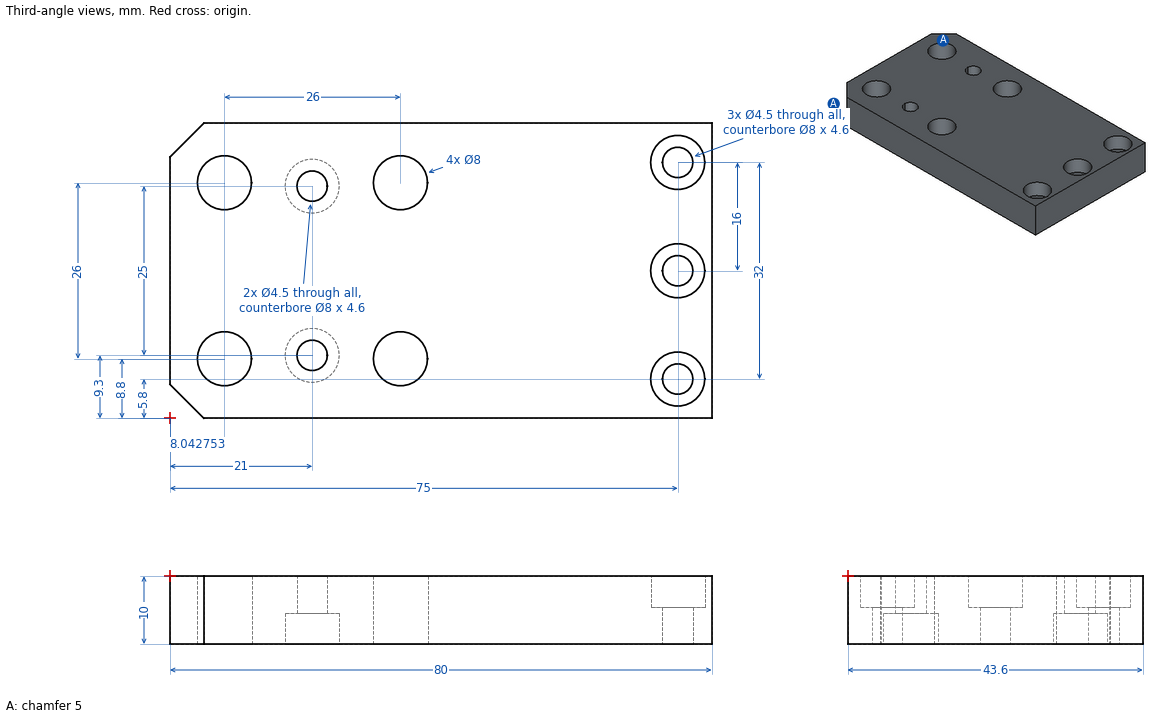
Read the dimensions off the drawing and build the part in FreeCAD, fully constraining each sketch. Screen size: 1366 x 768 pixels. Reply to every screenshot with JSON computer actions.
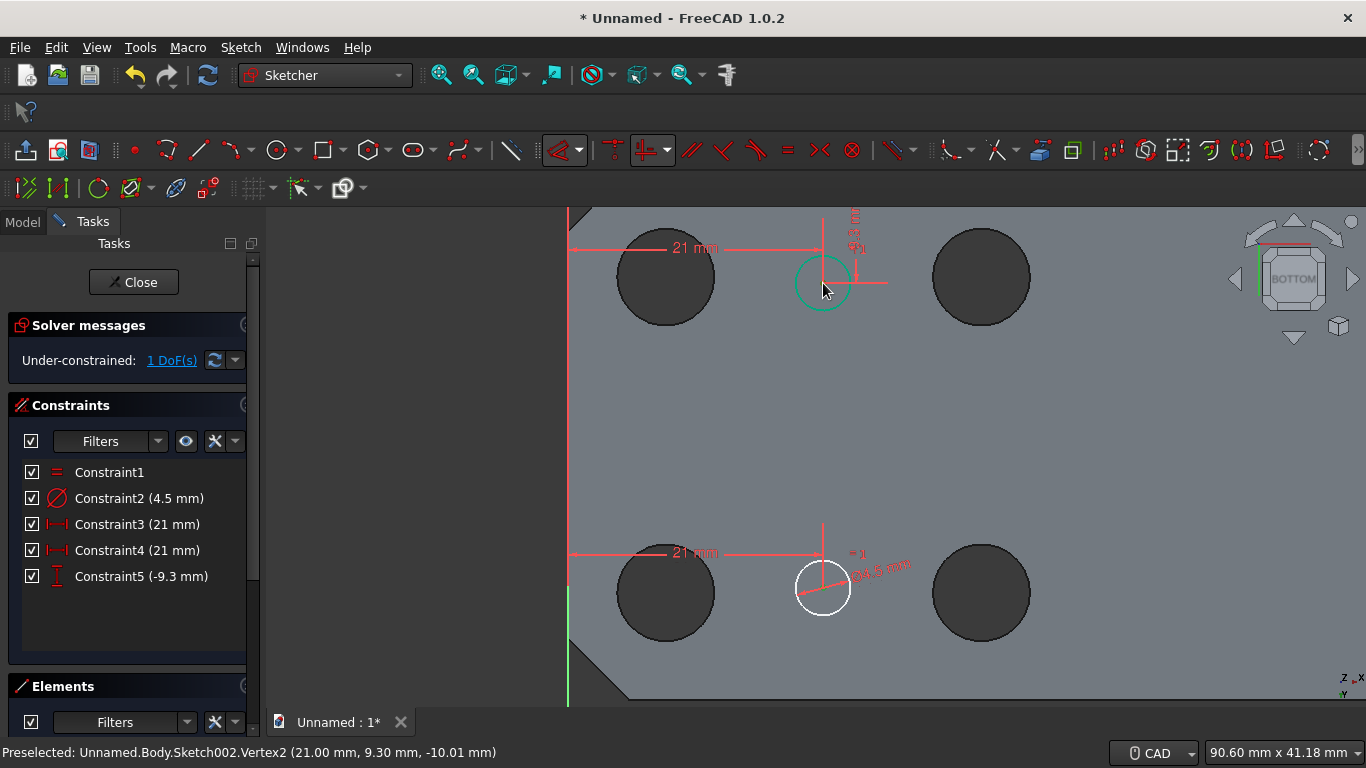
{"action": "key", "text": "i"}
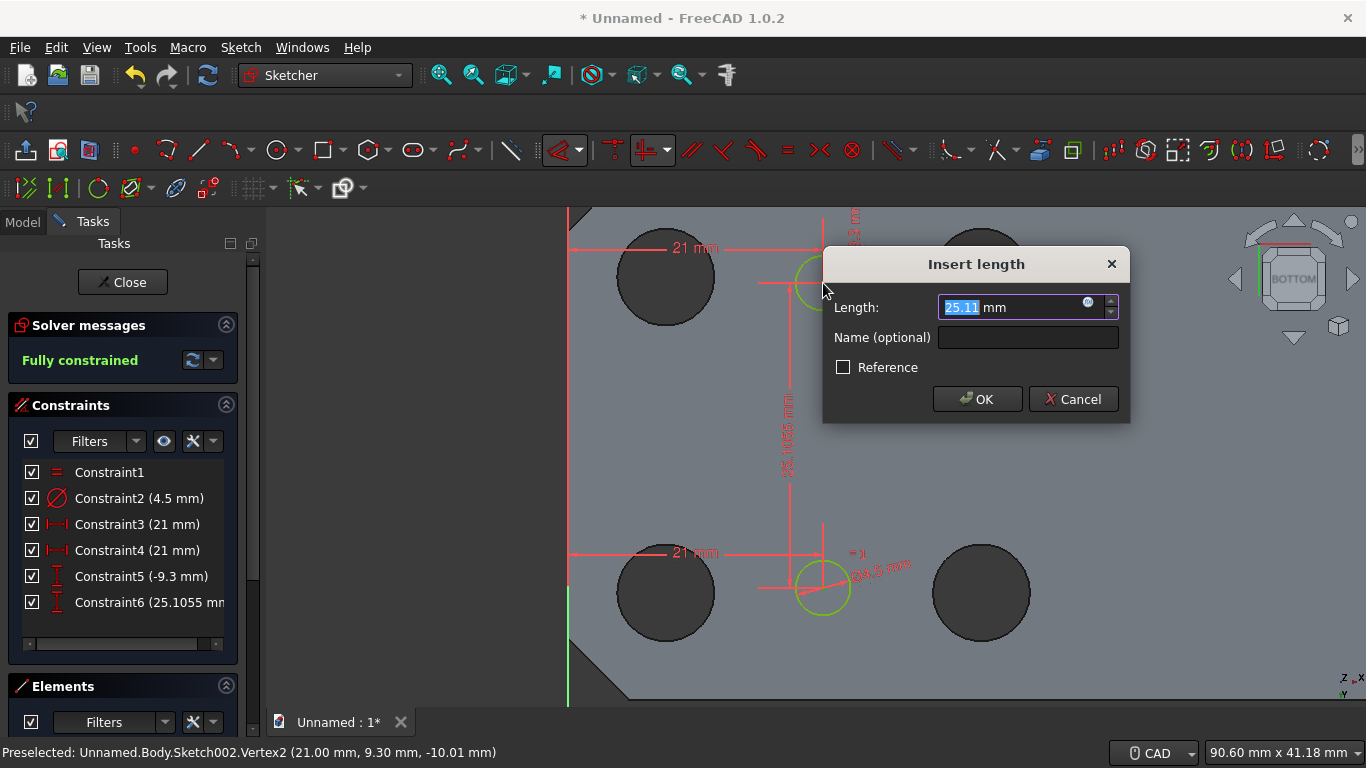
{"action": "type", "text": "25"}
{"action": "key", "text": "Return"}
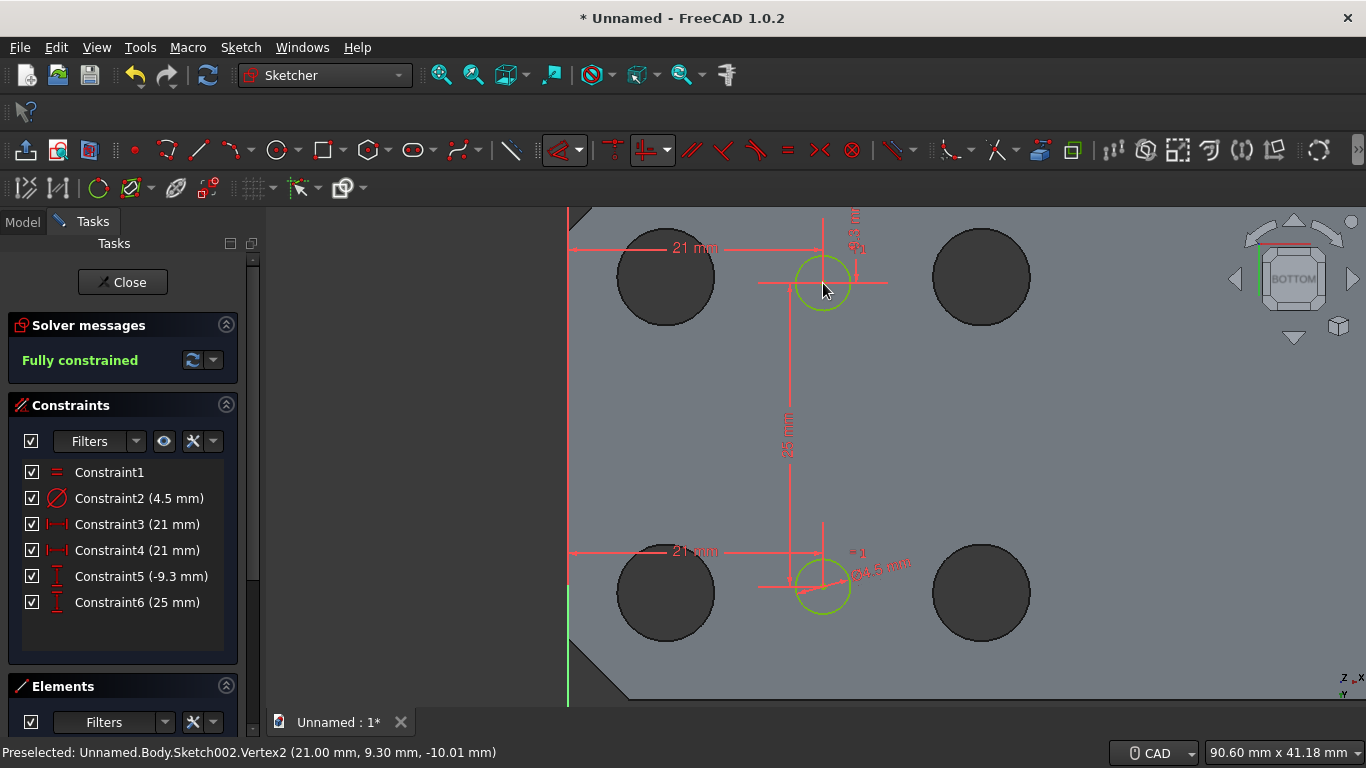
{"action": "left_click", "coordinate": [123, 282]}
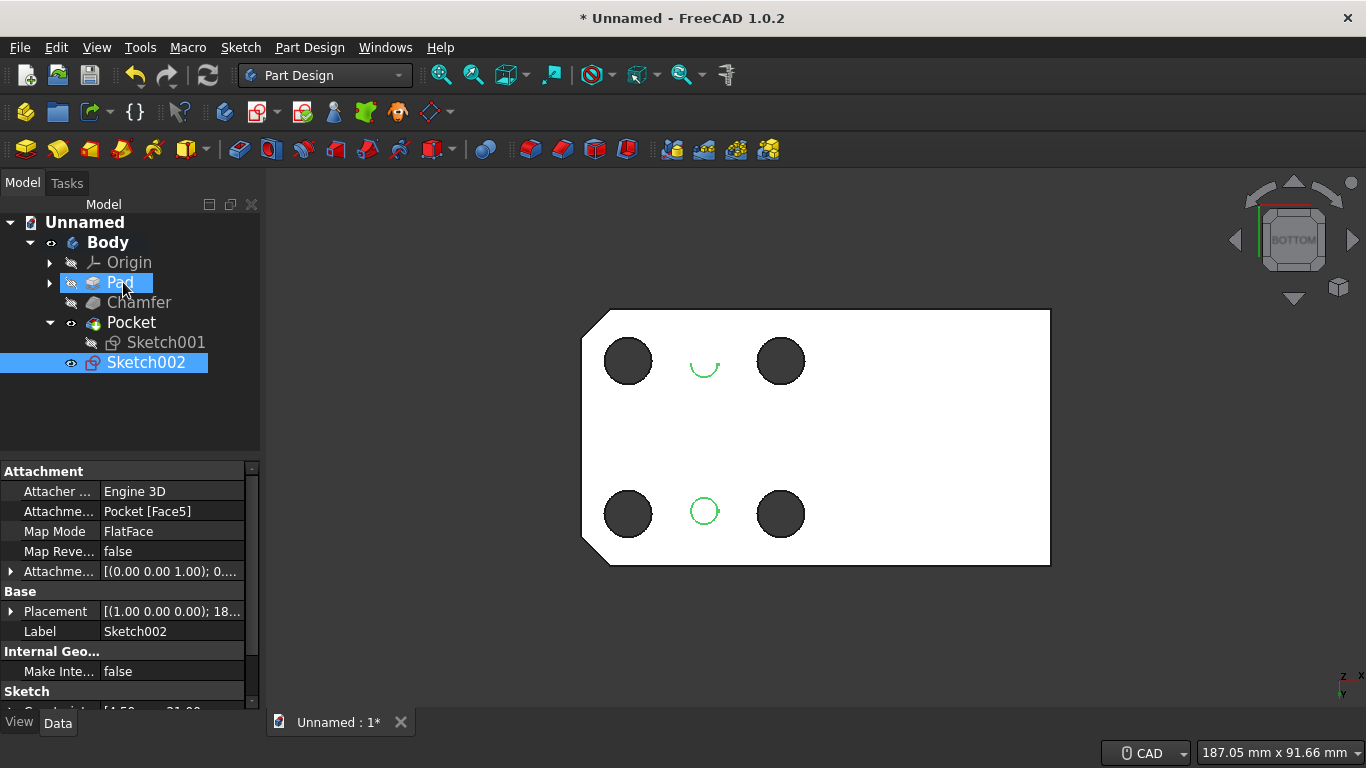
{"action": "left_click", "coordinate": [272, 150]}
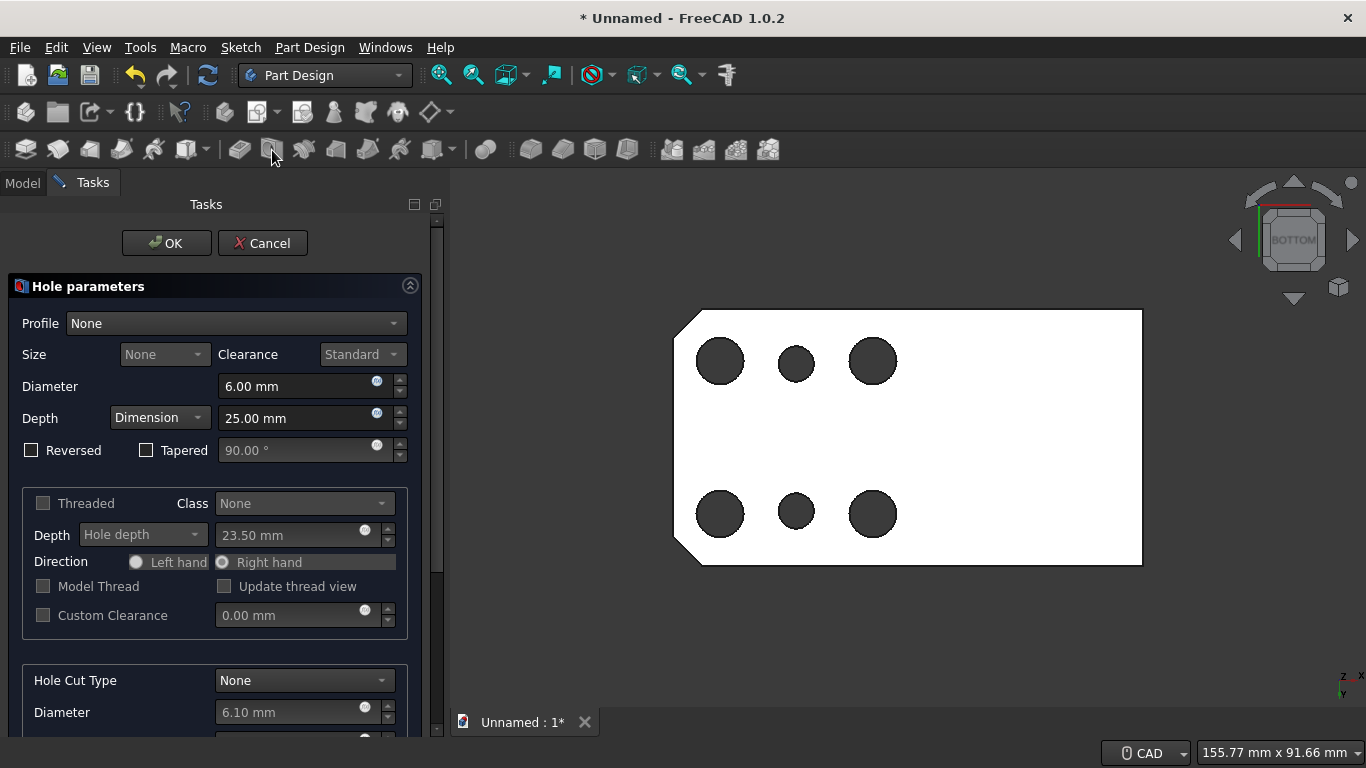
{"action": "triple_click", "coordinate": [305, 386]}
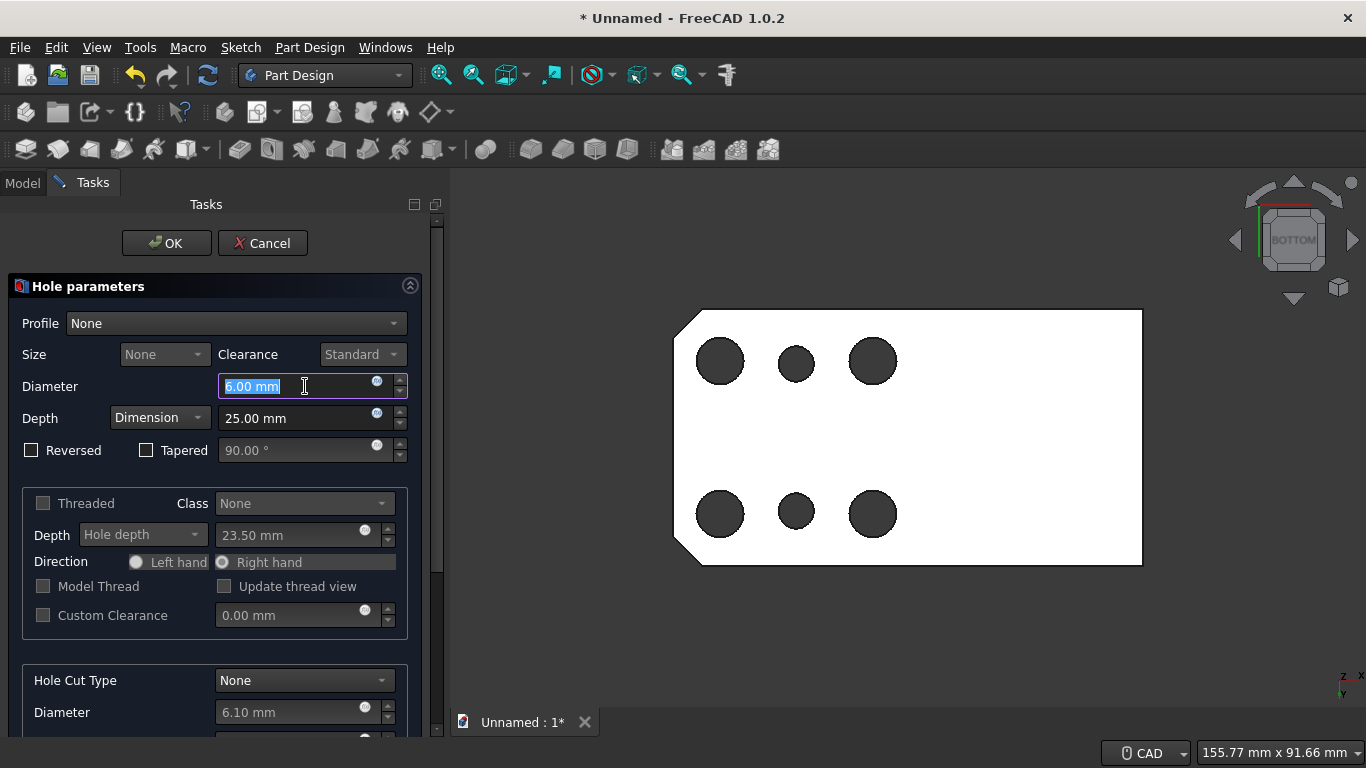
{"action": "type", "text": "4.5"}
{"action": "key", "text": "Tab"}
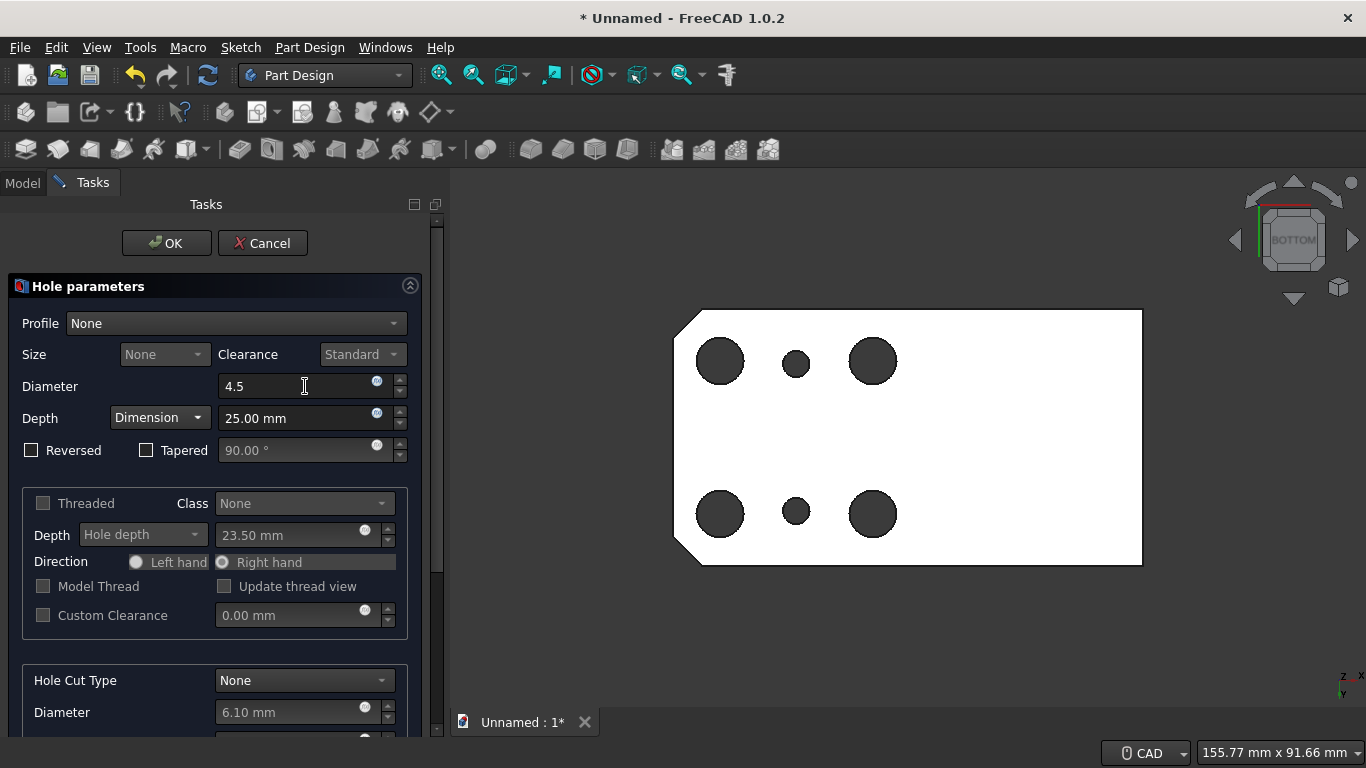
{"action": "left_click", "coordinate": [161, 418]}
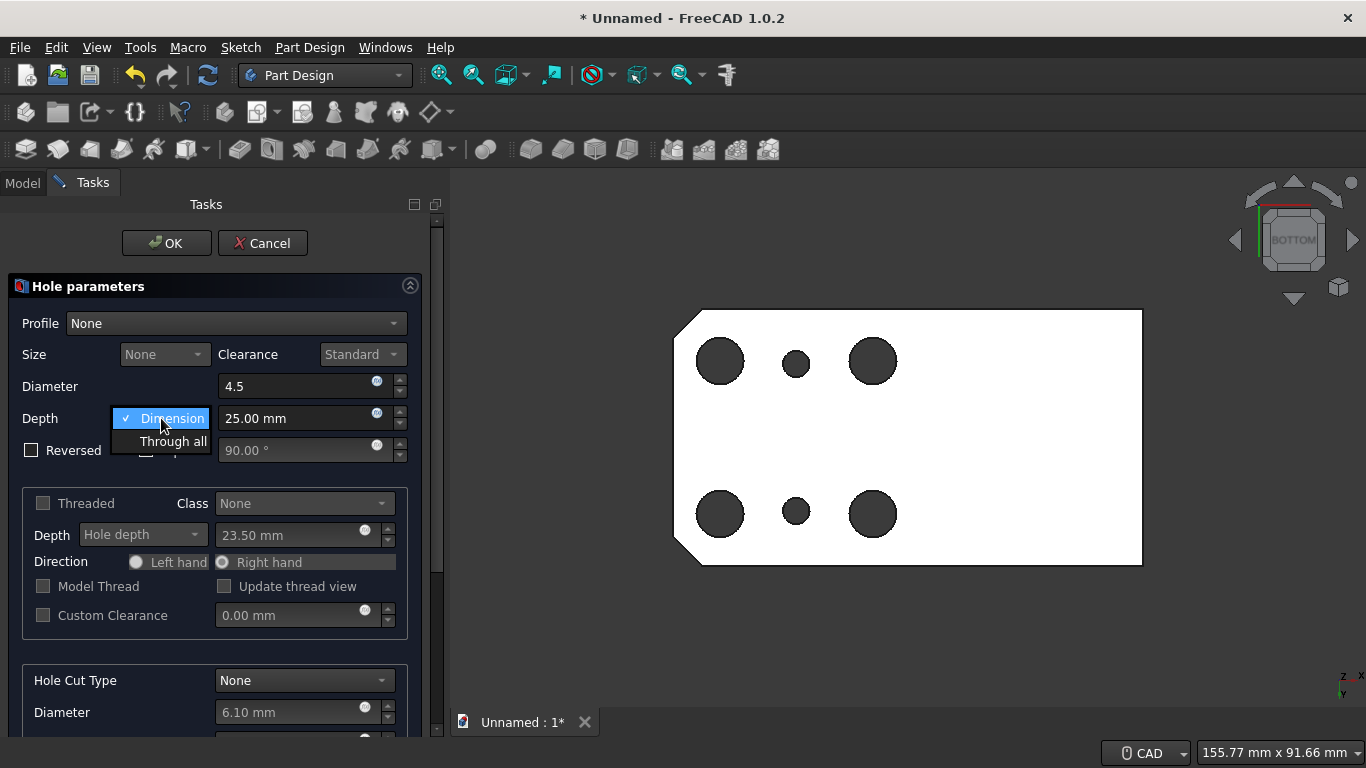
{"action": "left_click", "coordinate": [160, 442]}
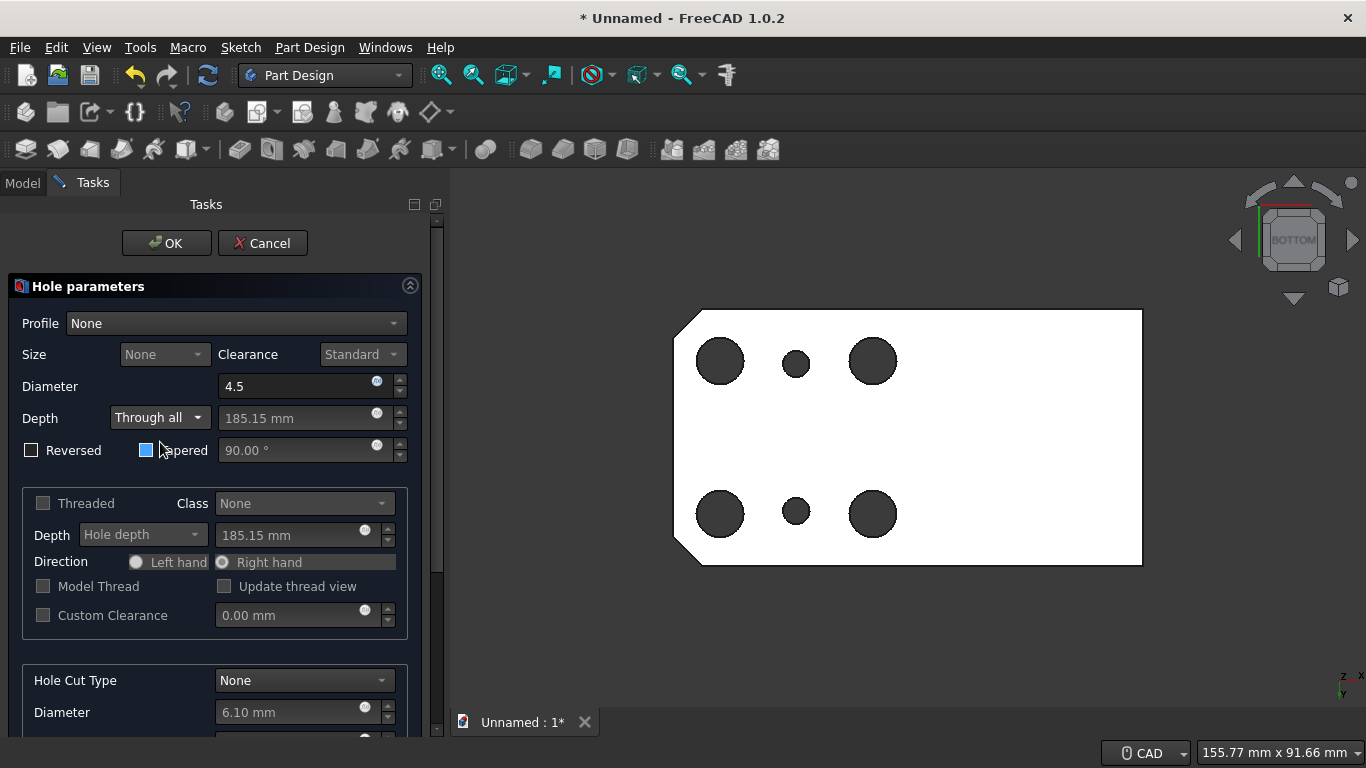
{"action": "left_click", "coordinate": [306, 680]}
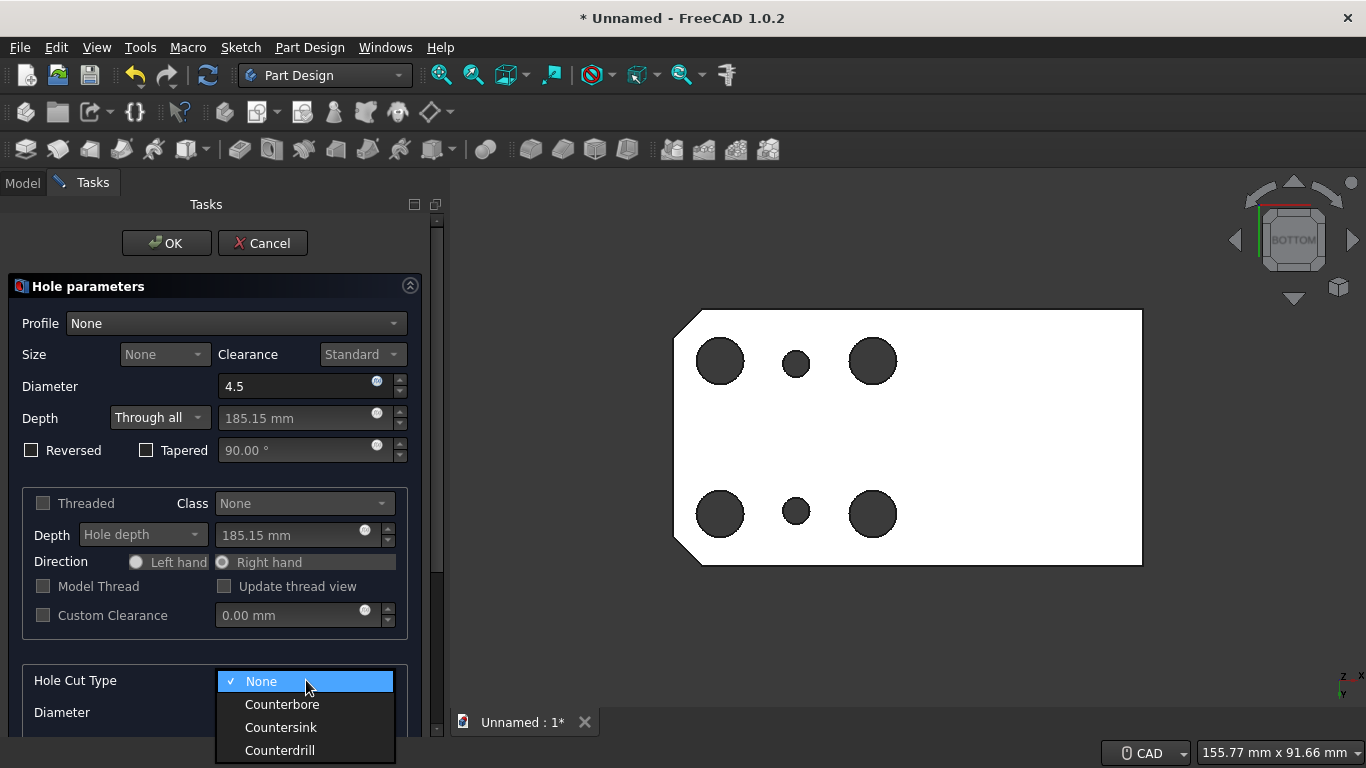
{"action": "left_click", "coordinate": [304, 704]}